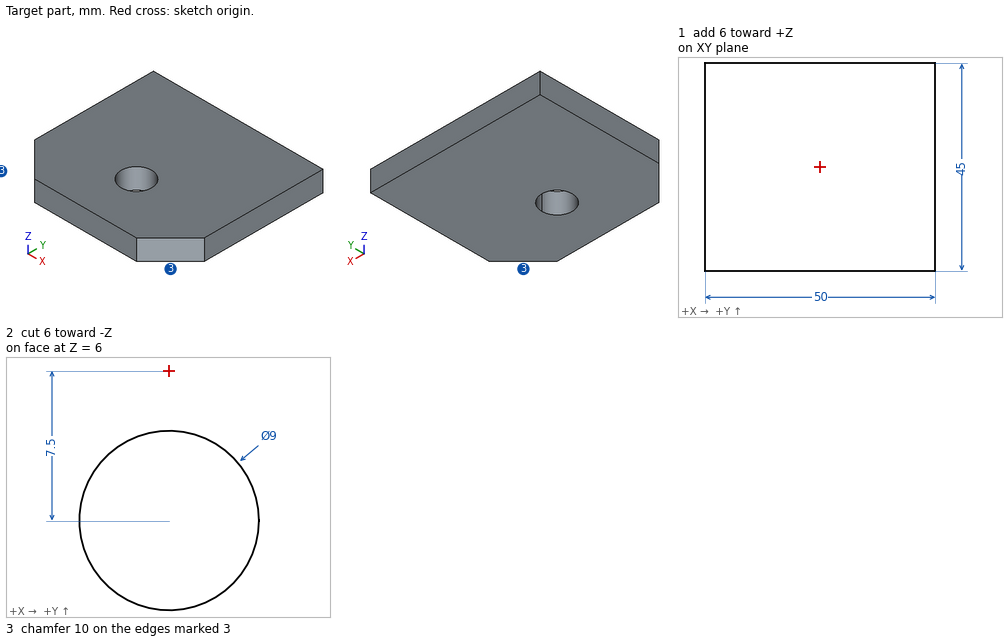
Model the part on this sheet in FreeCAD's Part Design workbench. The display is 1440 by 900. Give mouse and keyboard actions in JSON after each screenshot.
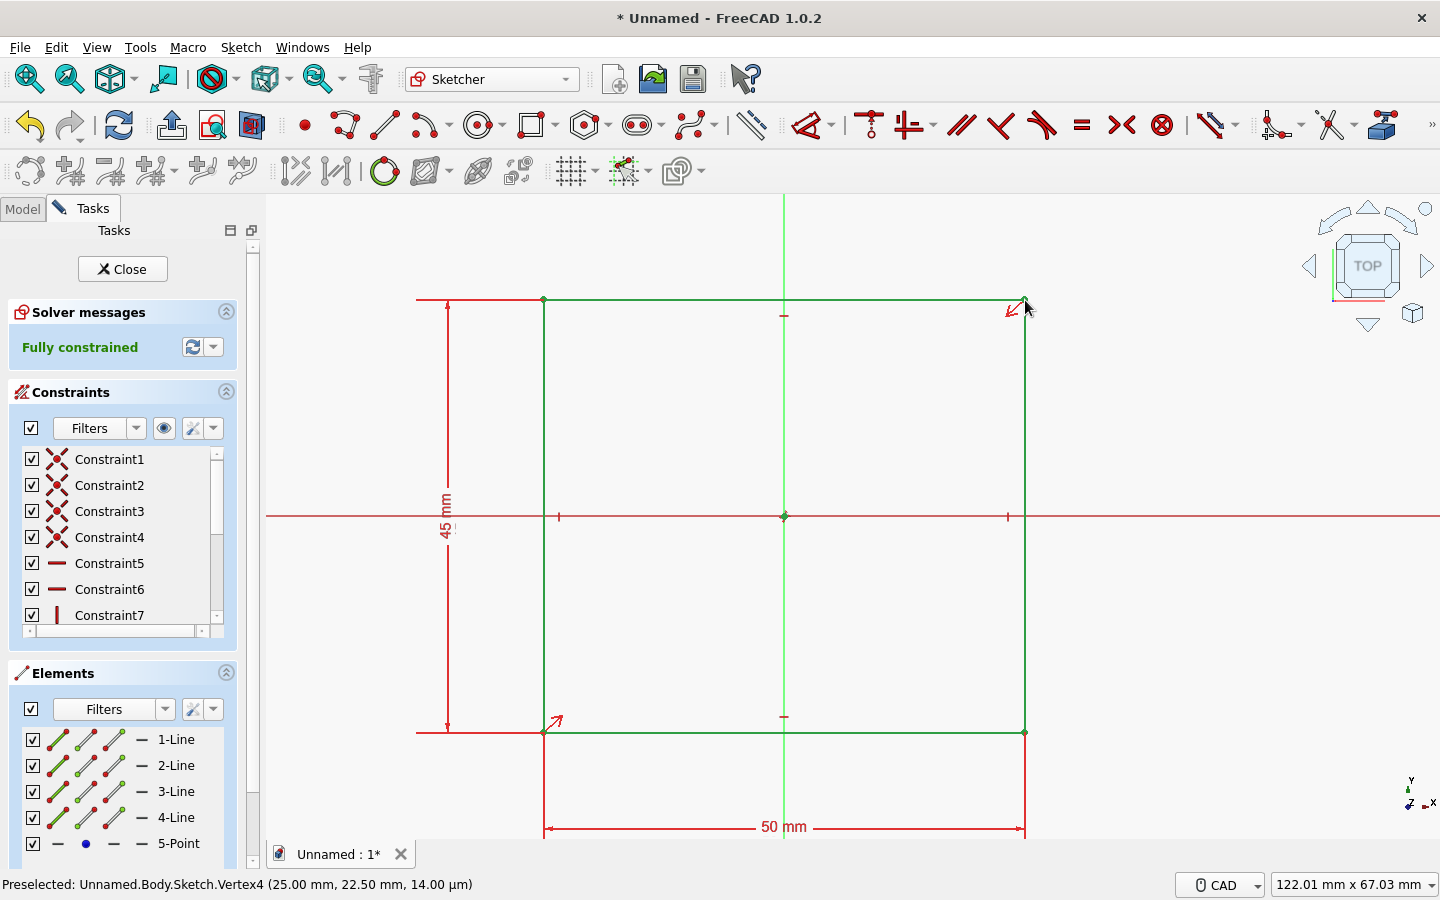
{"action": "left_click", "coordinate": [123, 269]}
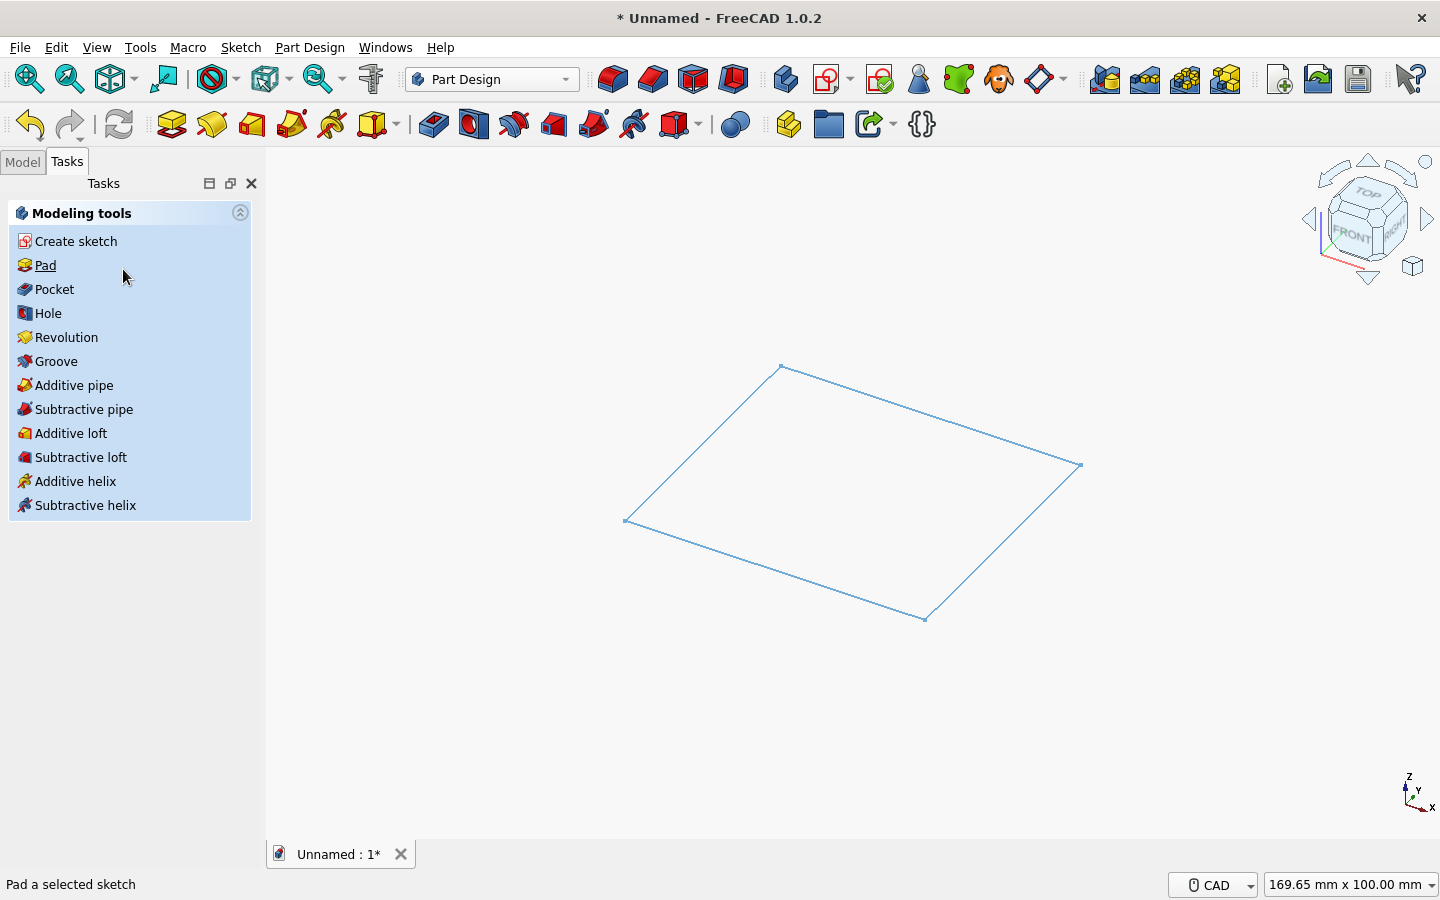
{"action": "left_click", "coordinate": [172, 124]}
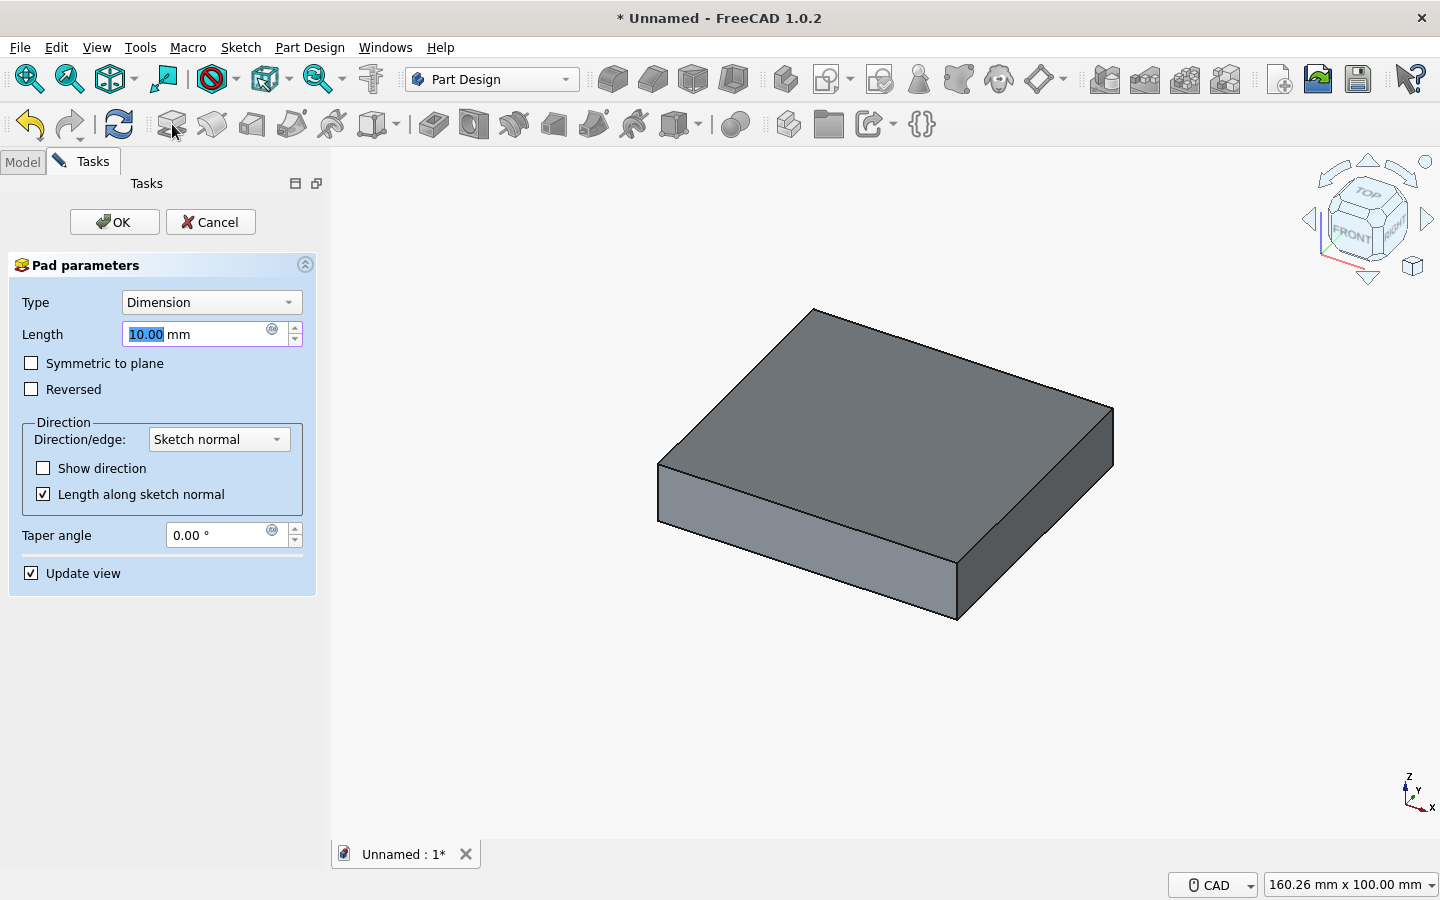
{"action": "type", "text": "6"}
{"action": "key", "text": "Tab"}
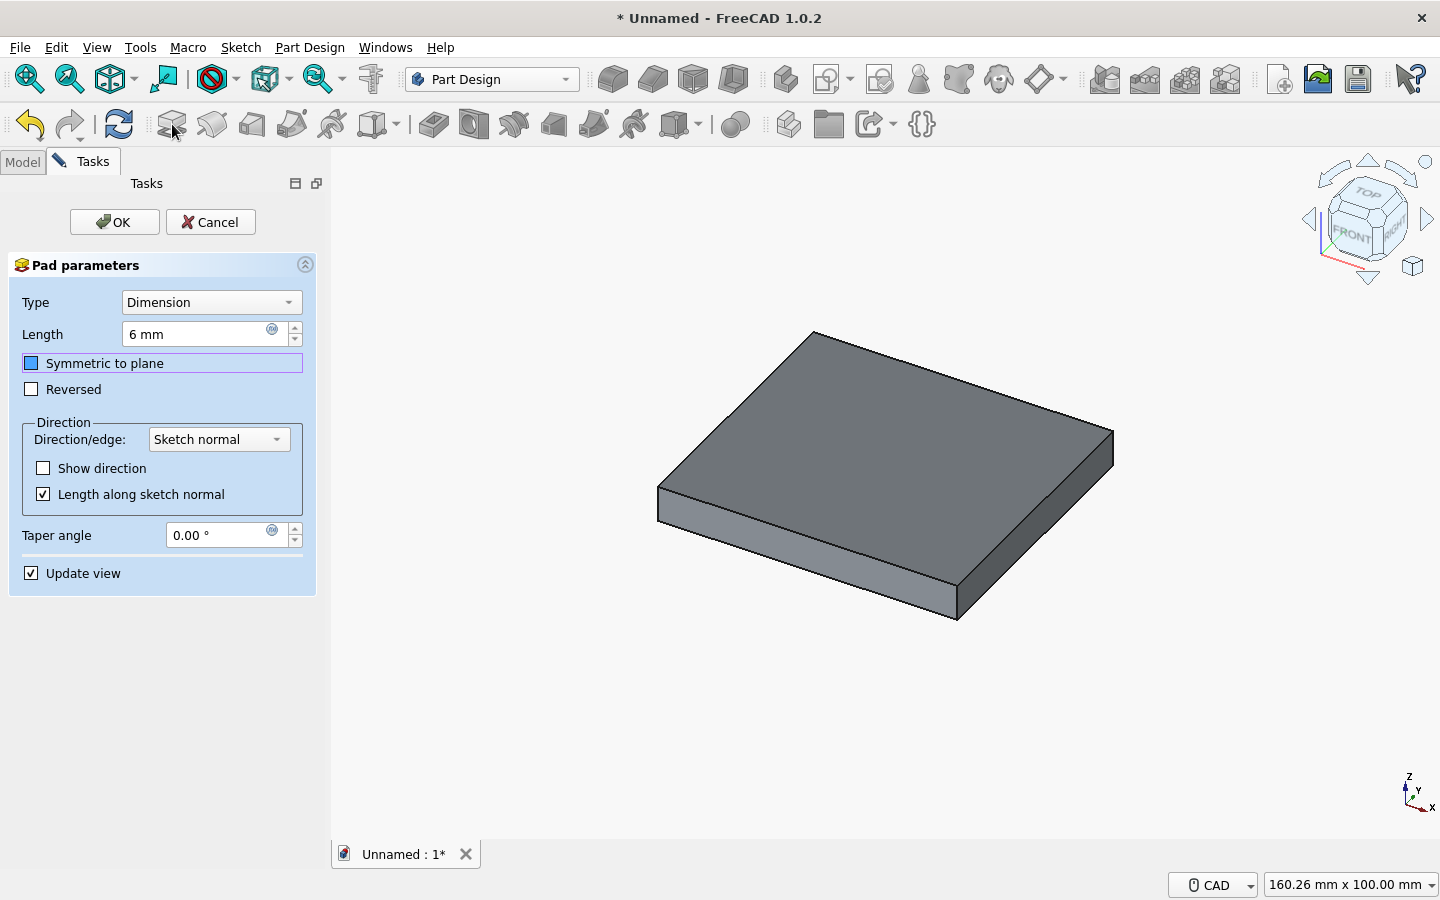
{"action": "left_click", "coordinate": [115, 222]}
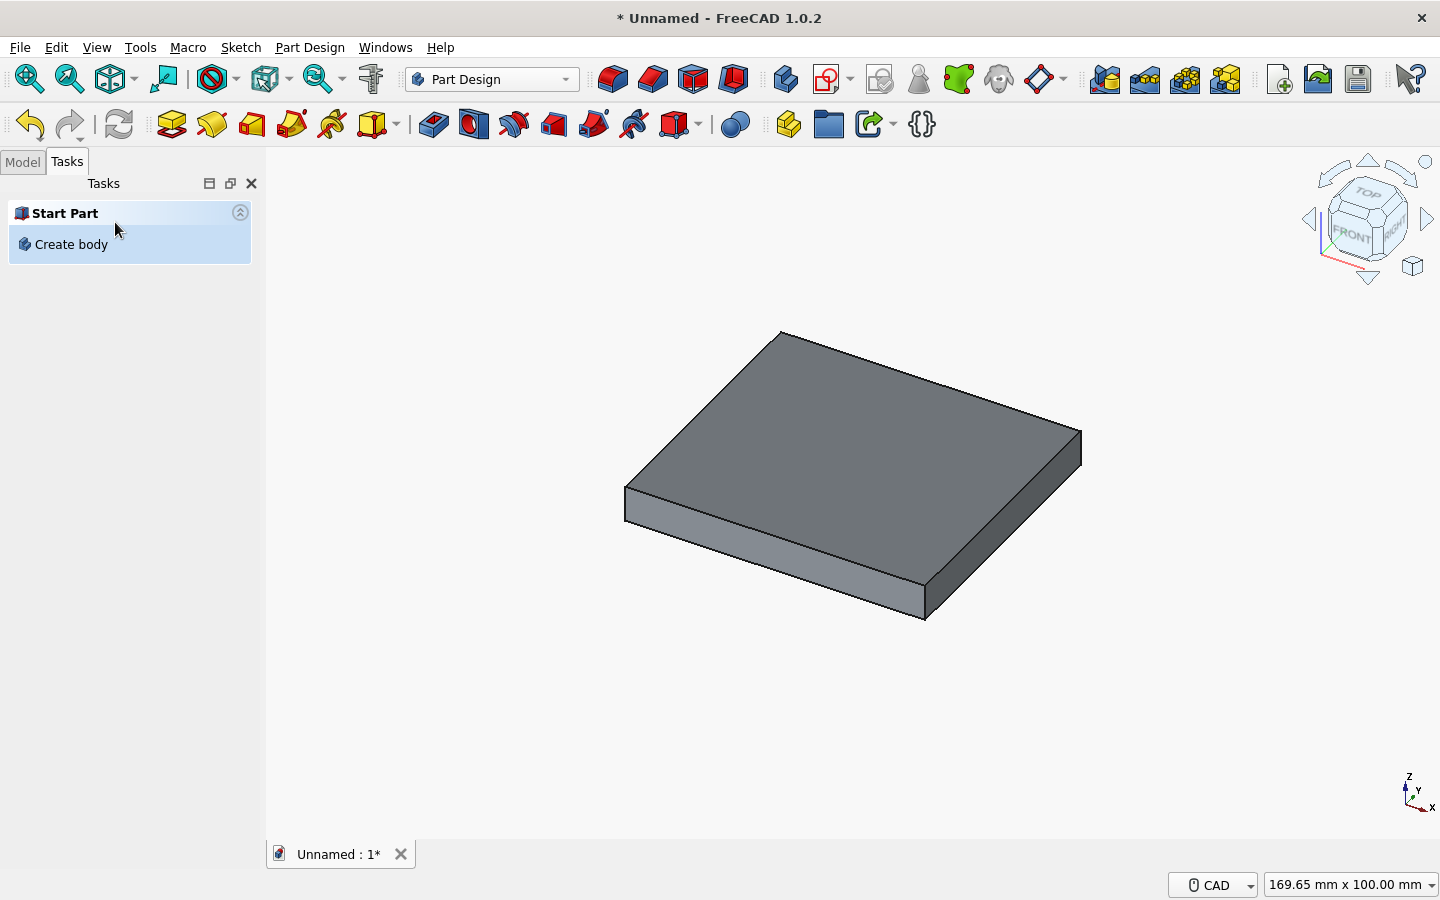
{"action": "key", "text": "v f"}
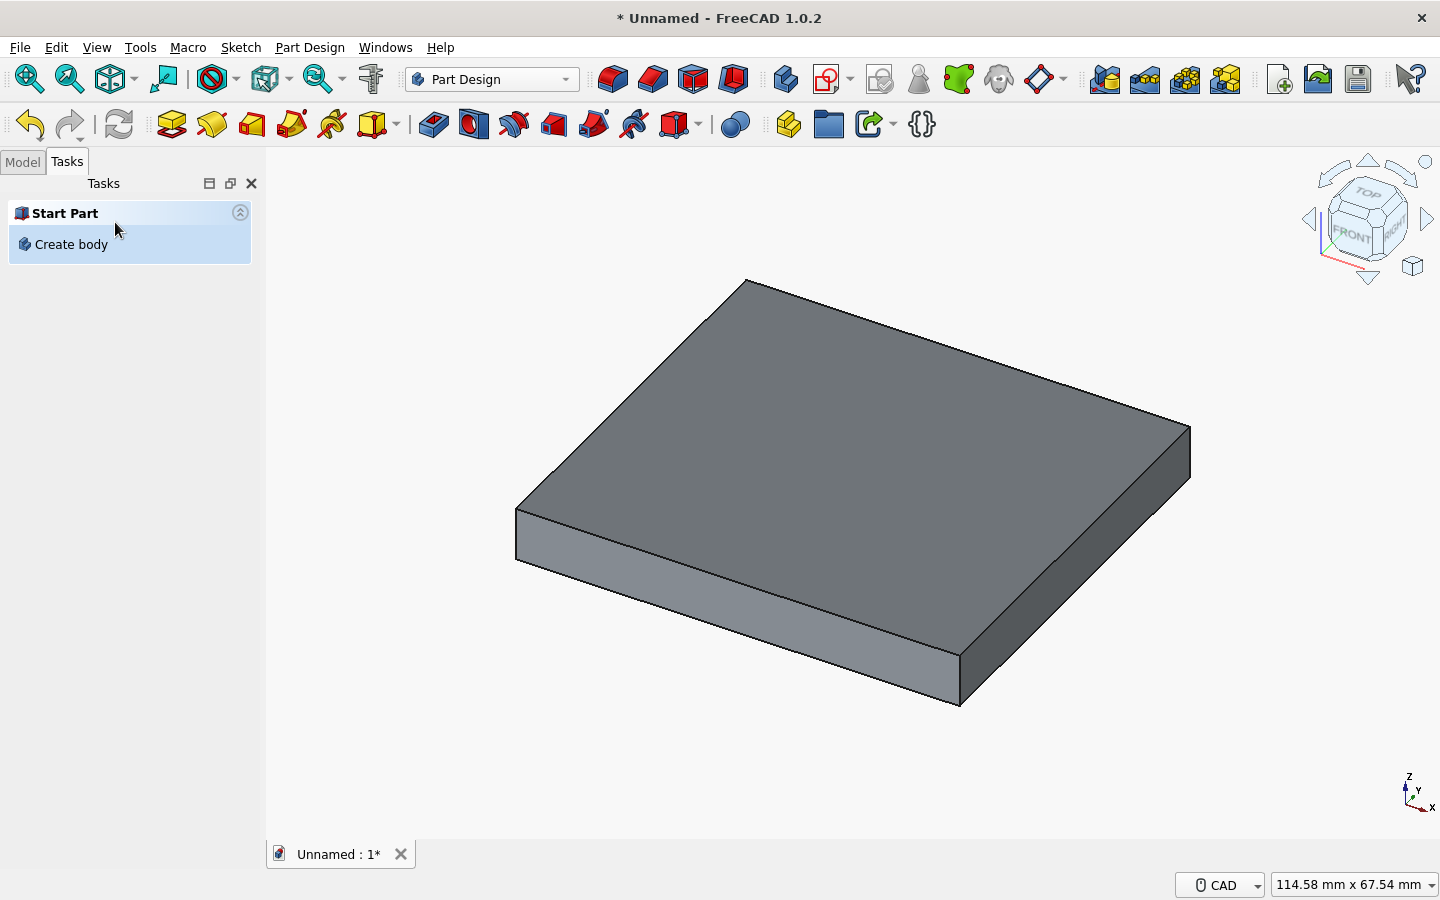
{"action": "left_click", "coordinate": [853, 467]}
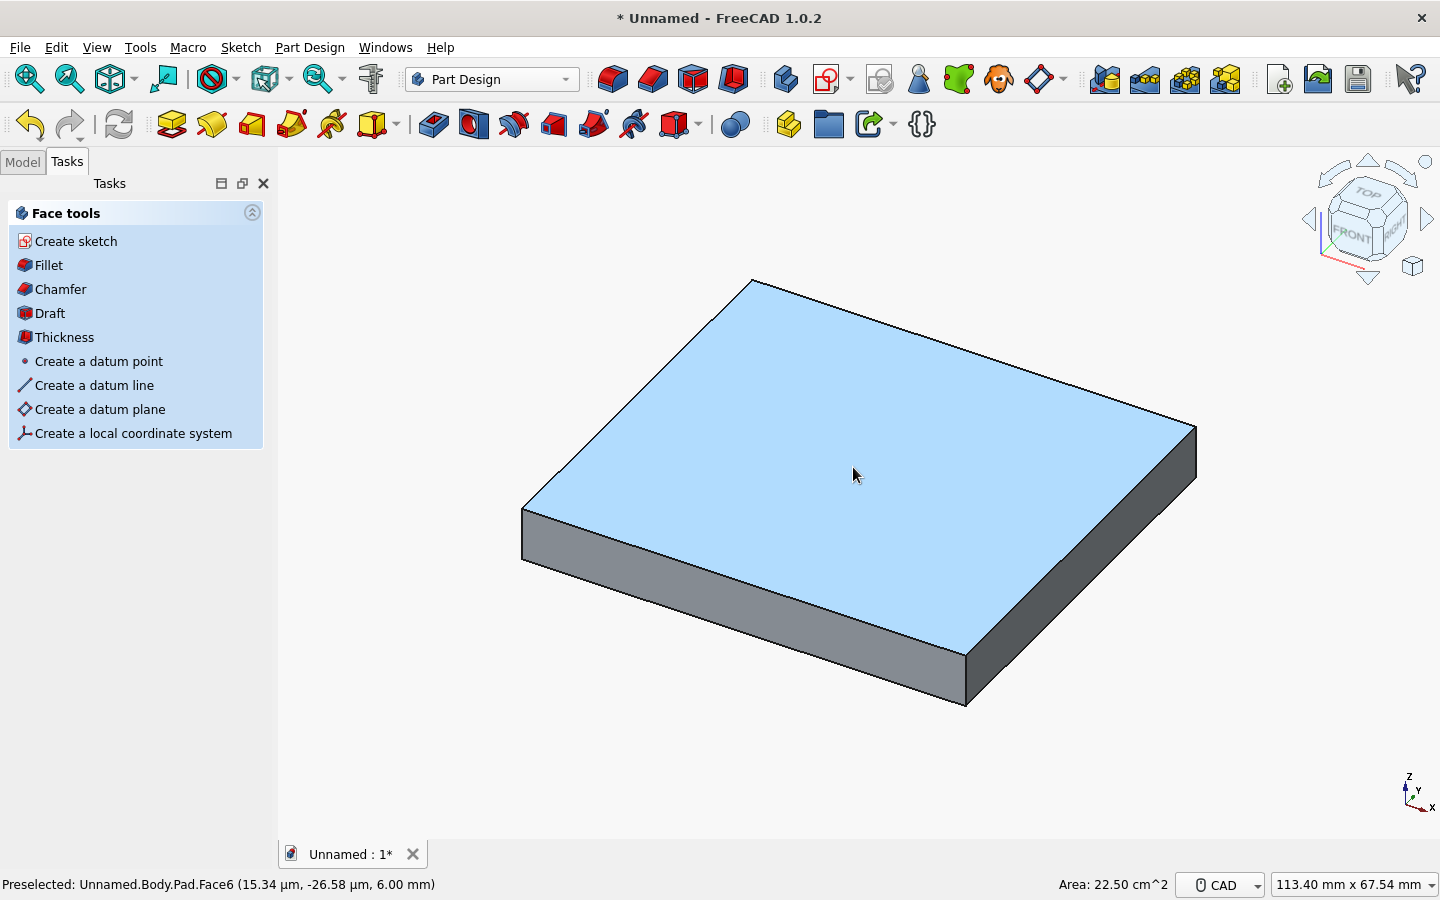
{"action": "left_click", "coordinate": [826, 80]}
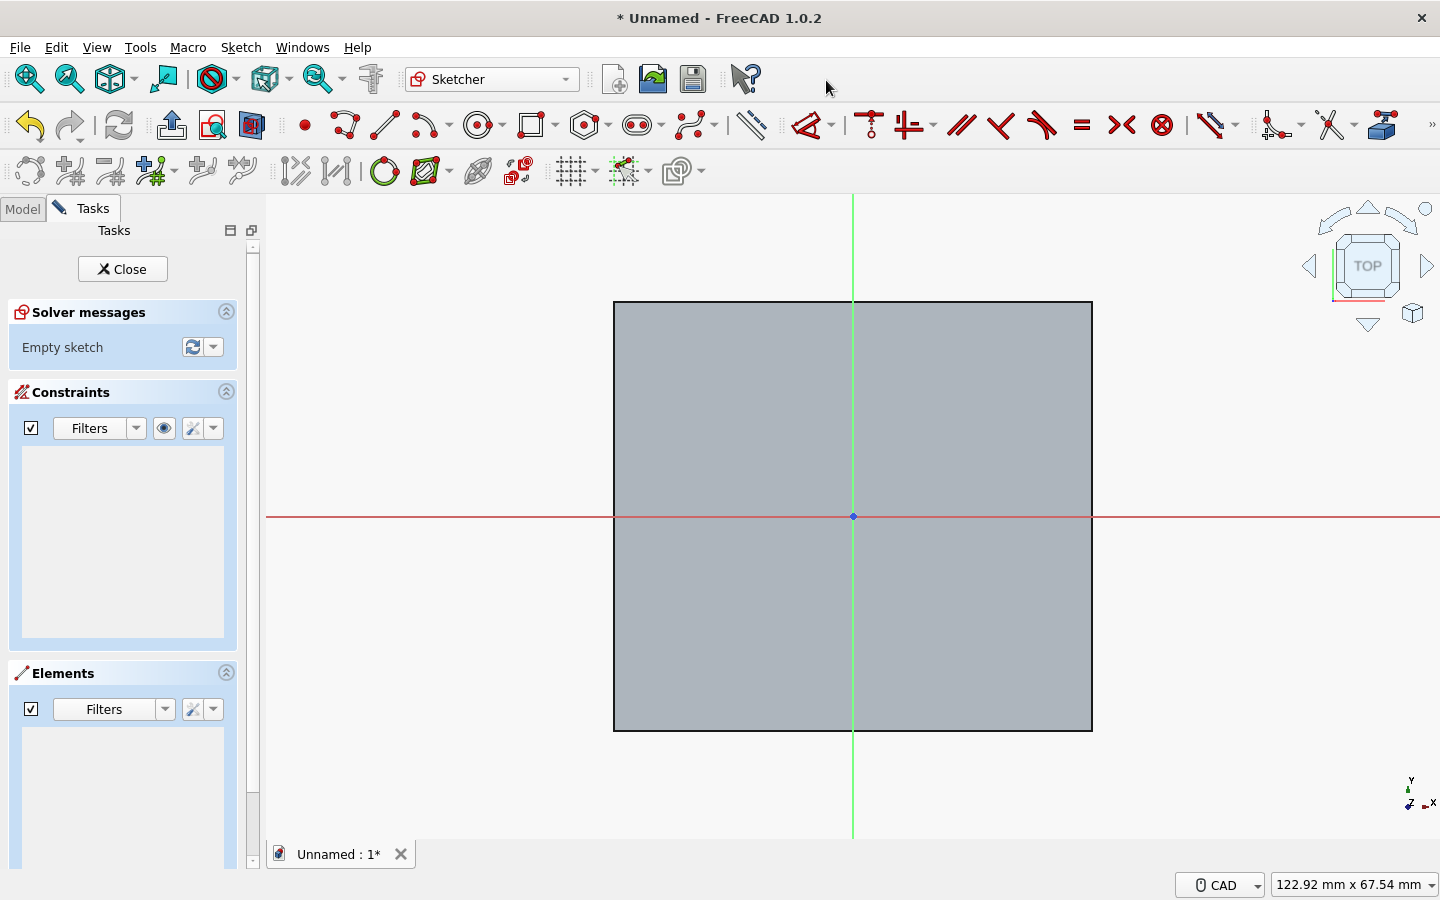
{"action": "scroll", "coordinate": [883, 599], "scroll_direction": "up", "scroll_amount": 6}